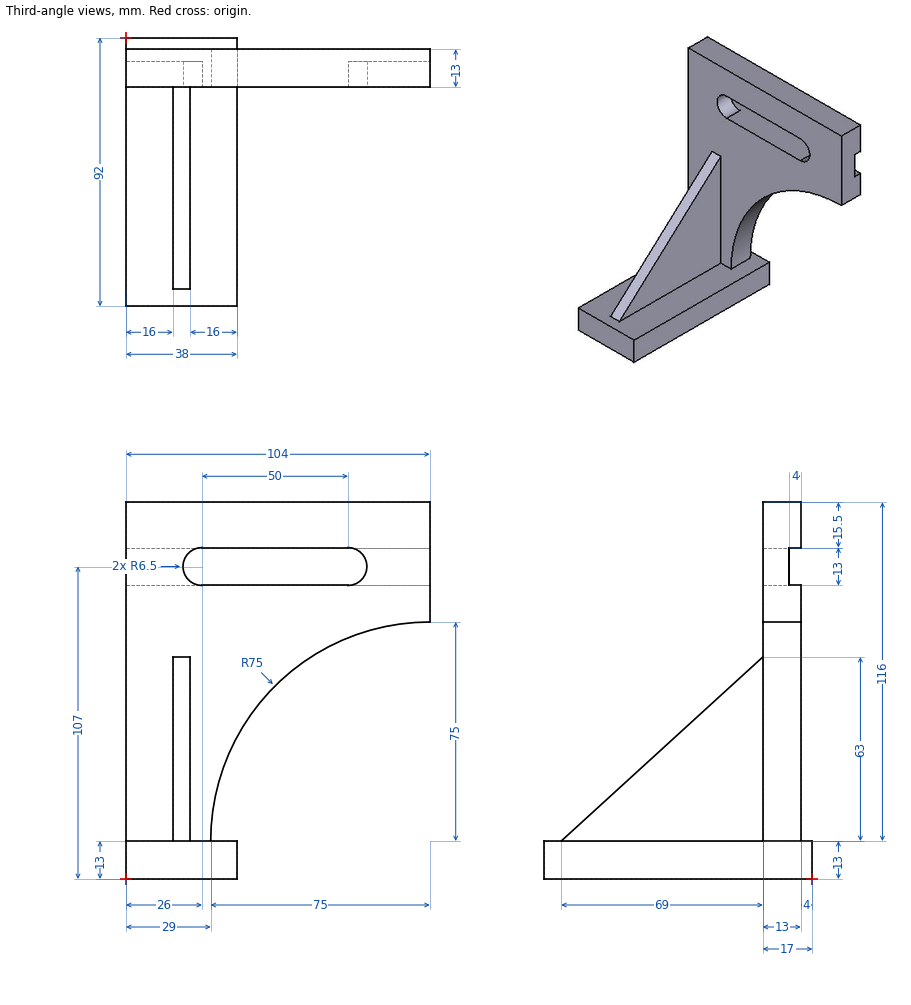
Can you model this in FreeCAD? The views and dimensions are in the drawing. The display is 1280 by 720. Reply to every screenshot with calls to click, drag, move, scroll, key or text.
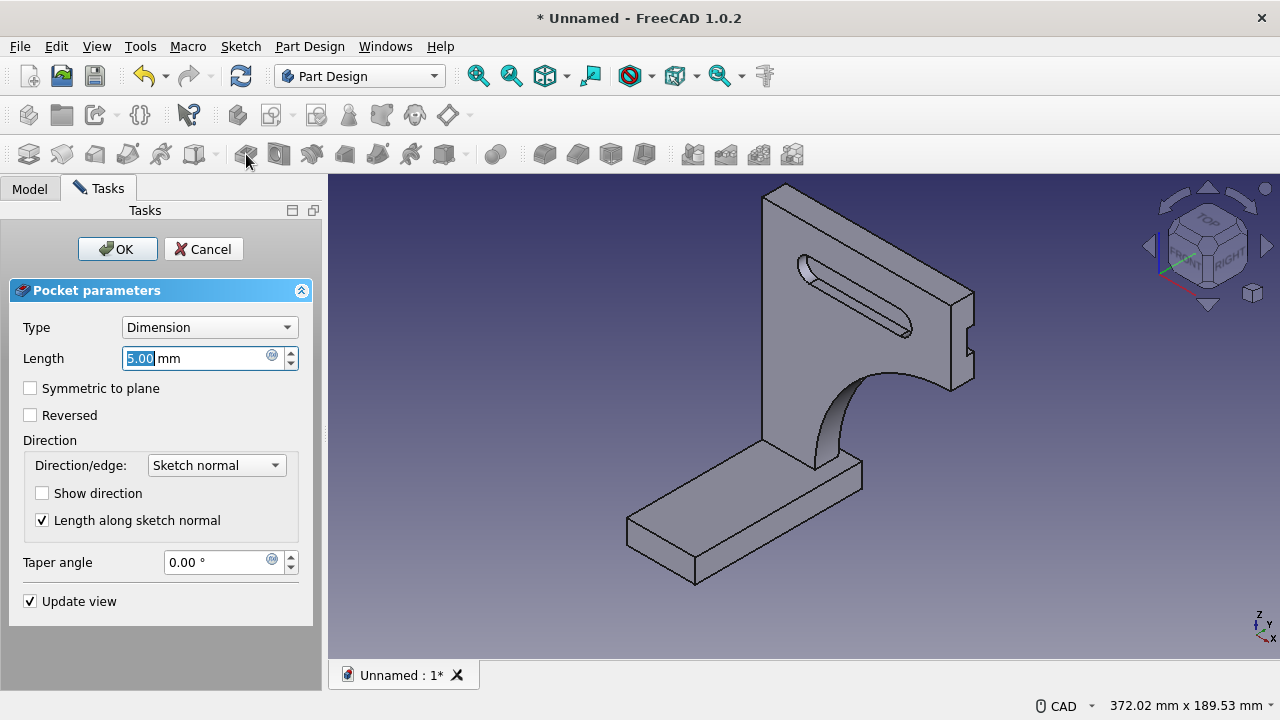
text(13)
key(Tab)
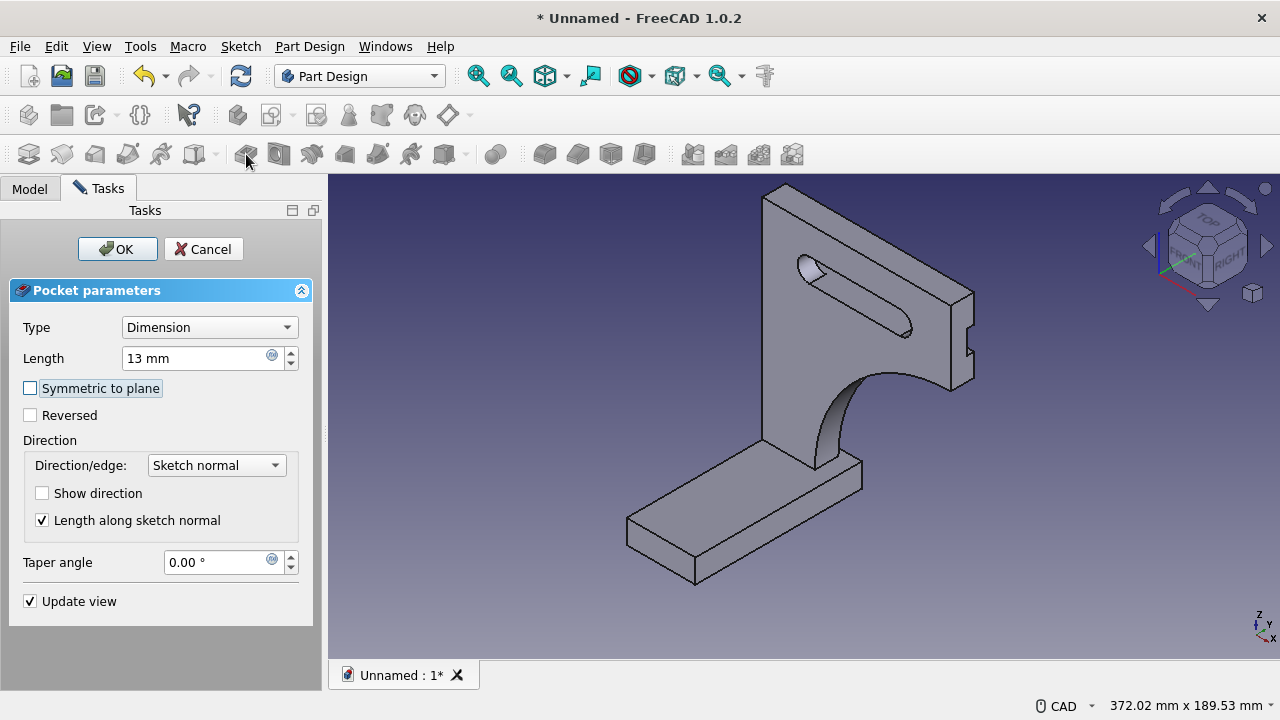
click(118, 249)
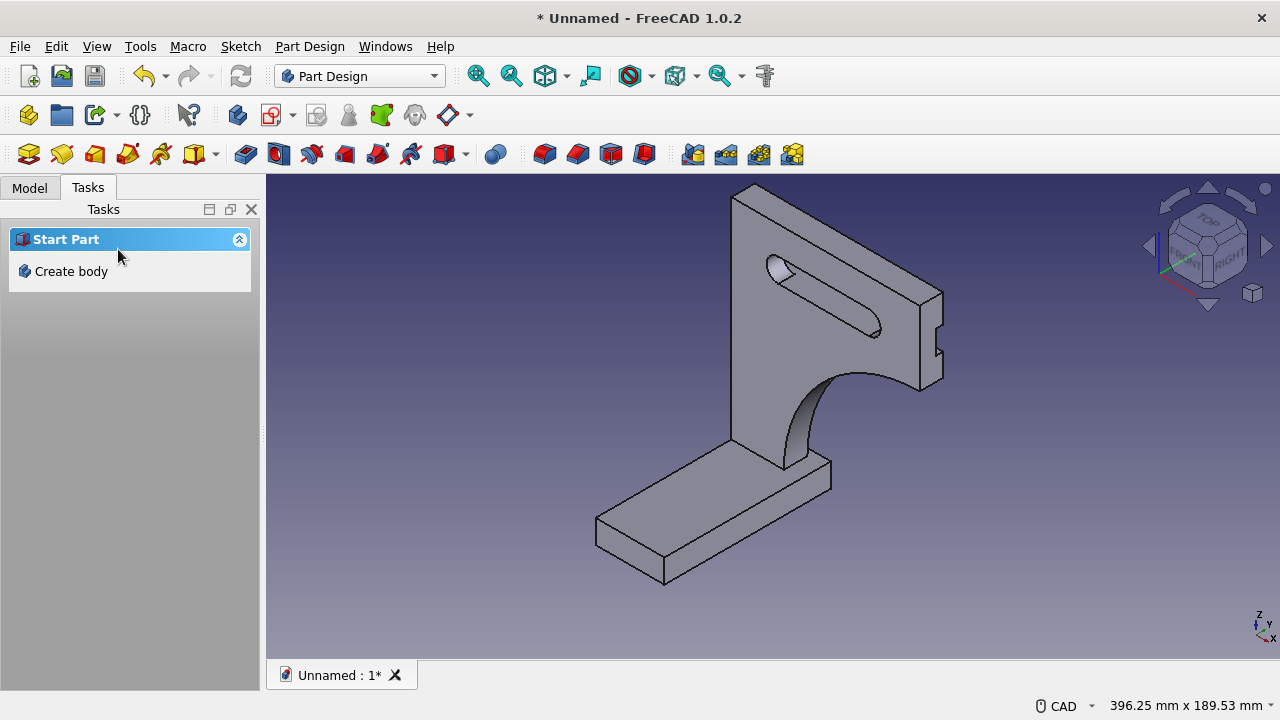
click(270, 116)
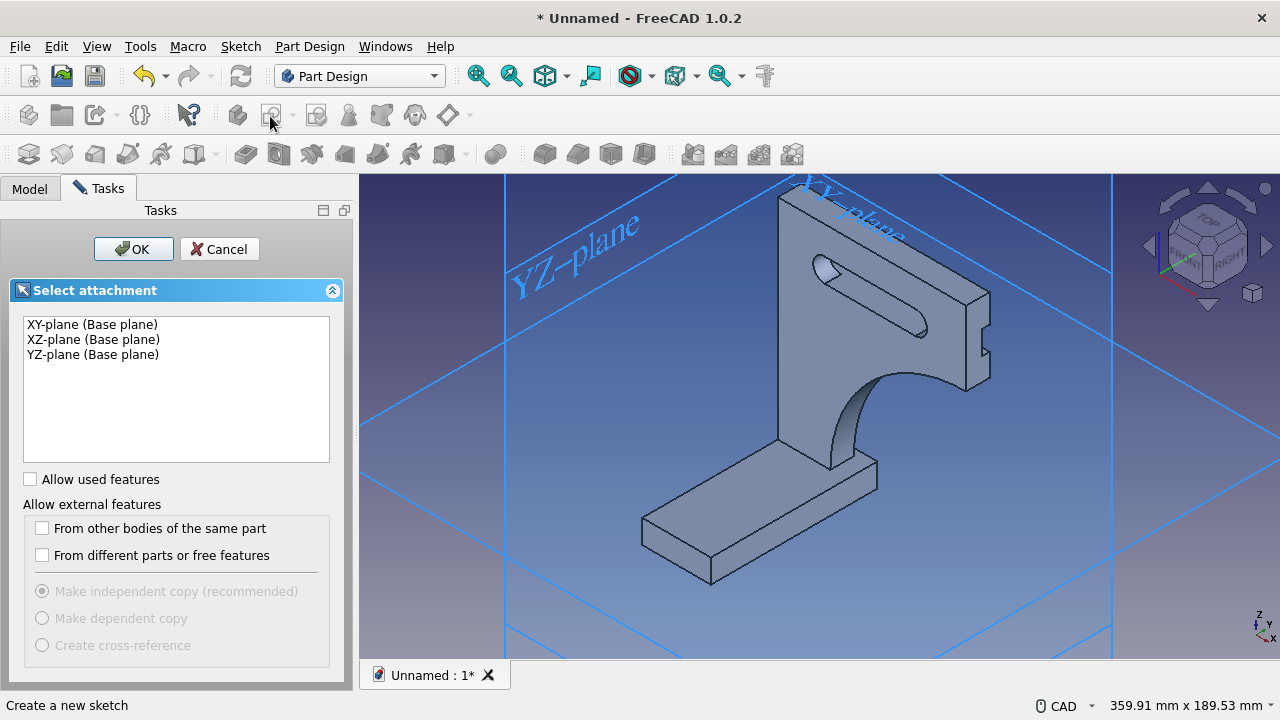
click(84, 354)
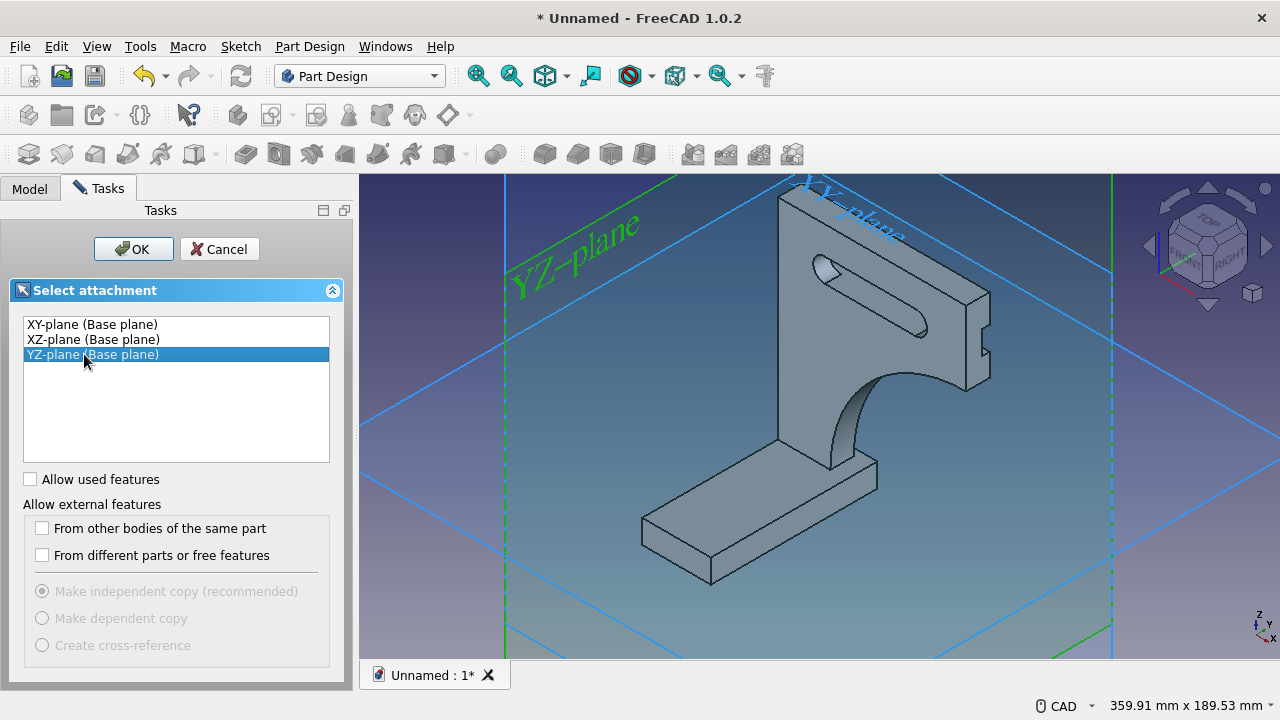
click(134, 249)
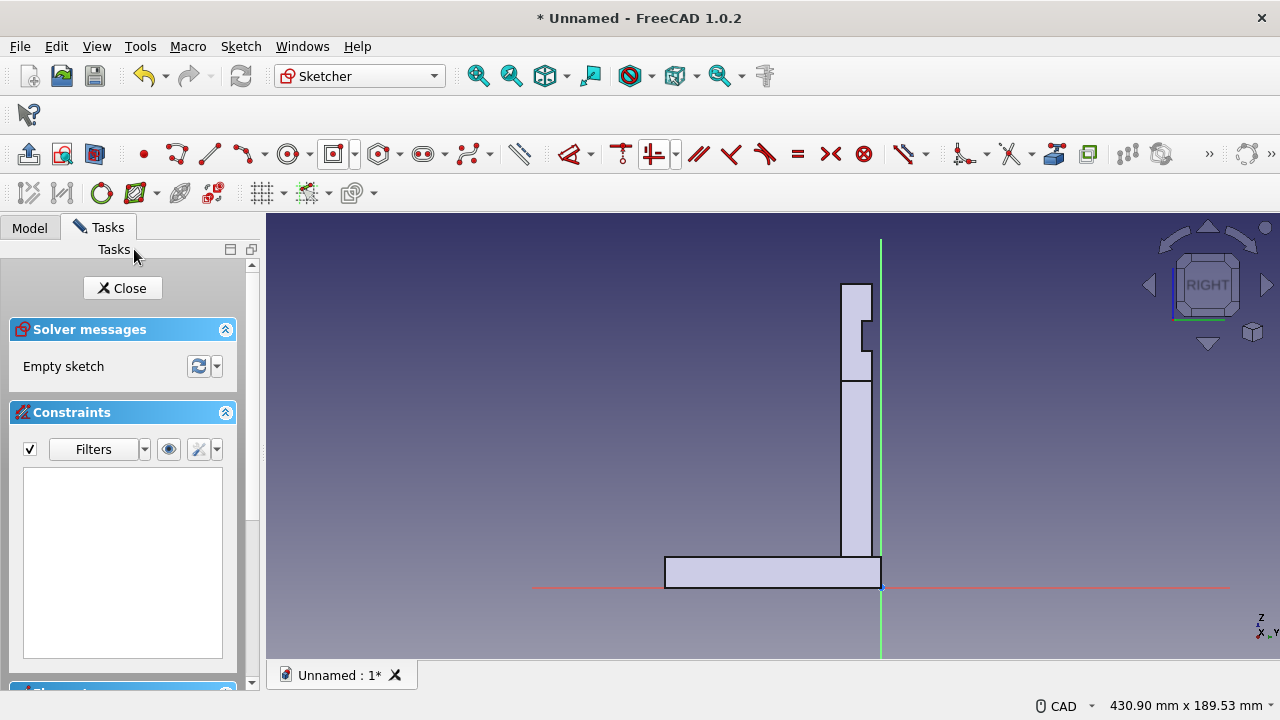
click(95, 154)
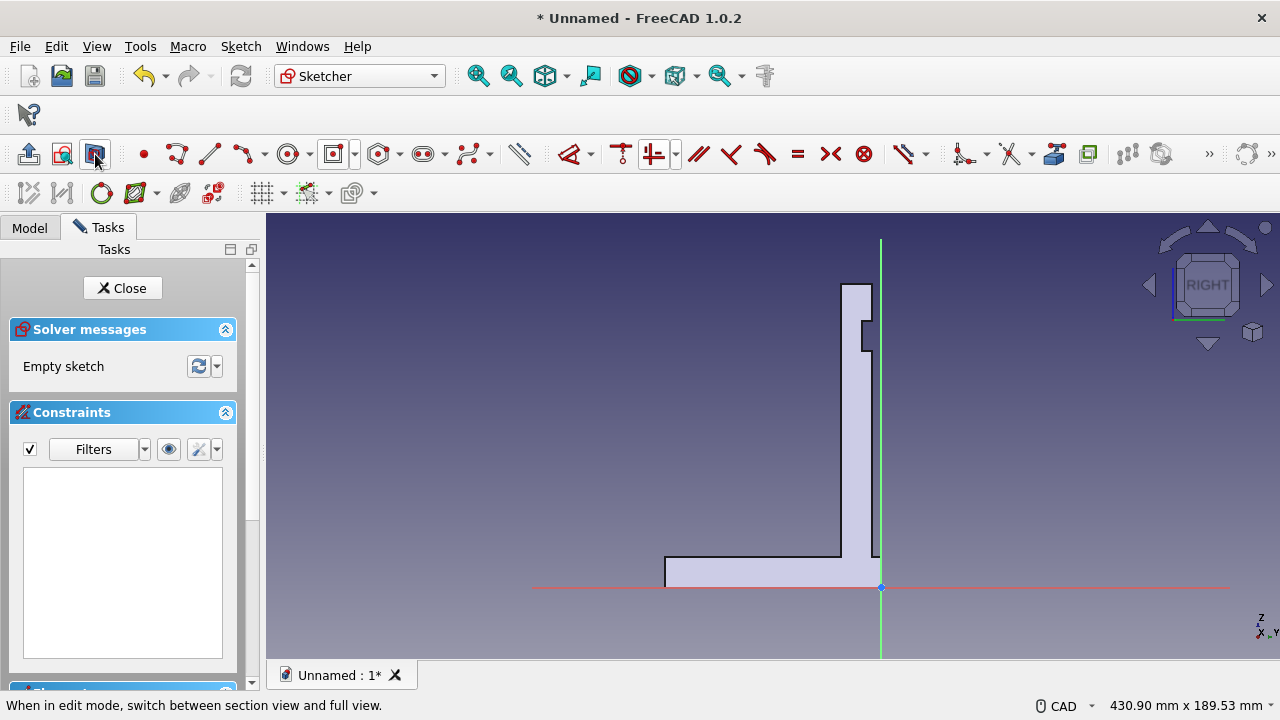
scroll(934, 625, up, 2)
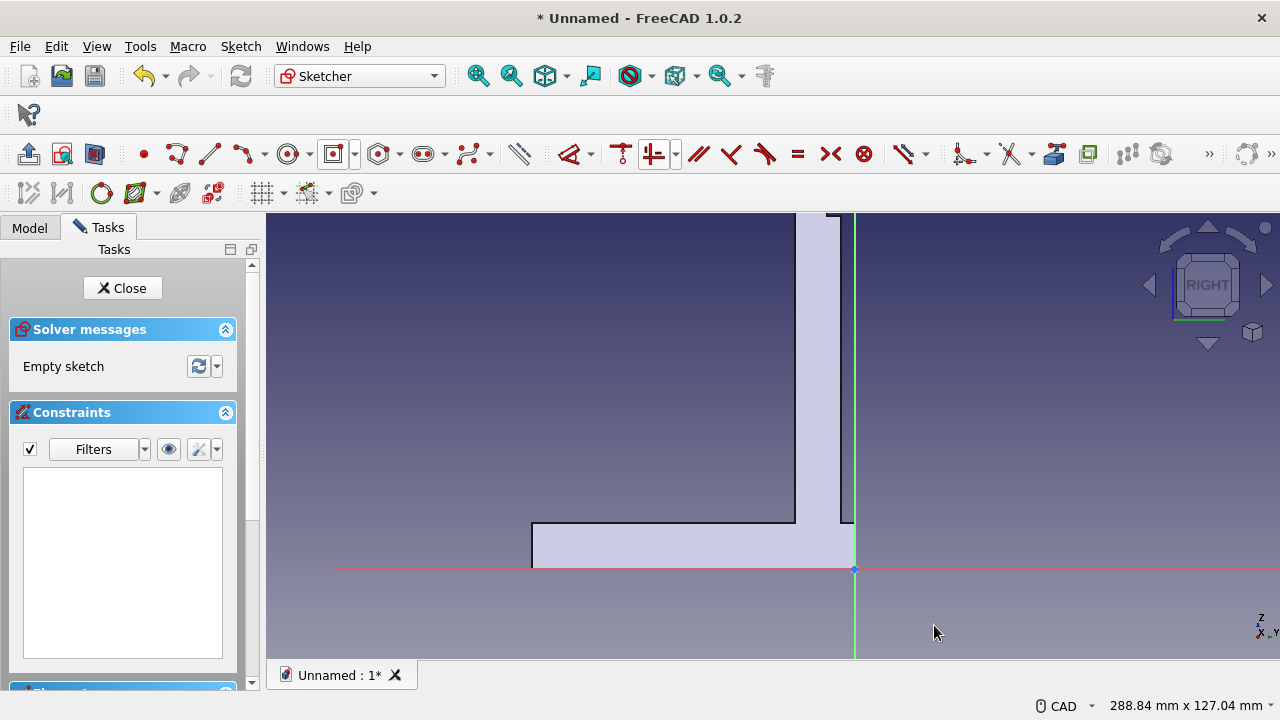
click(177, 154)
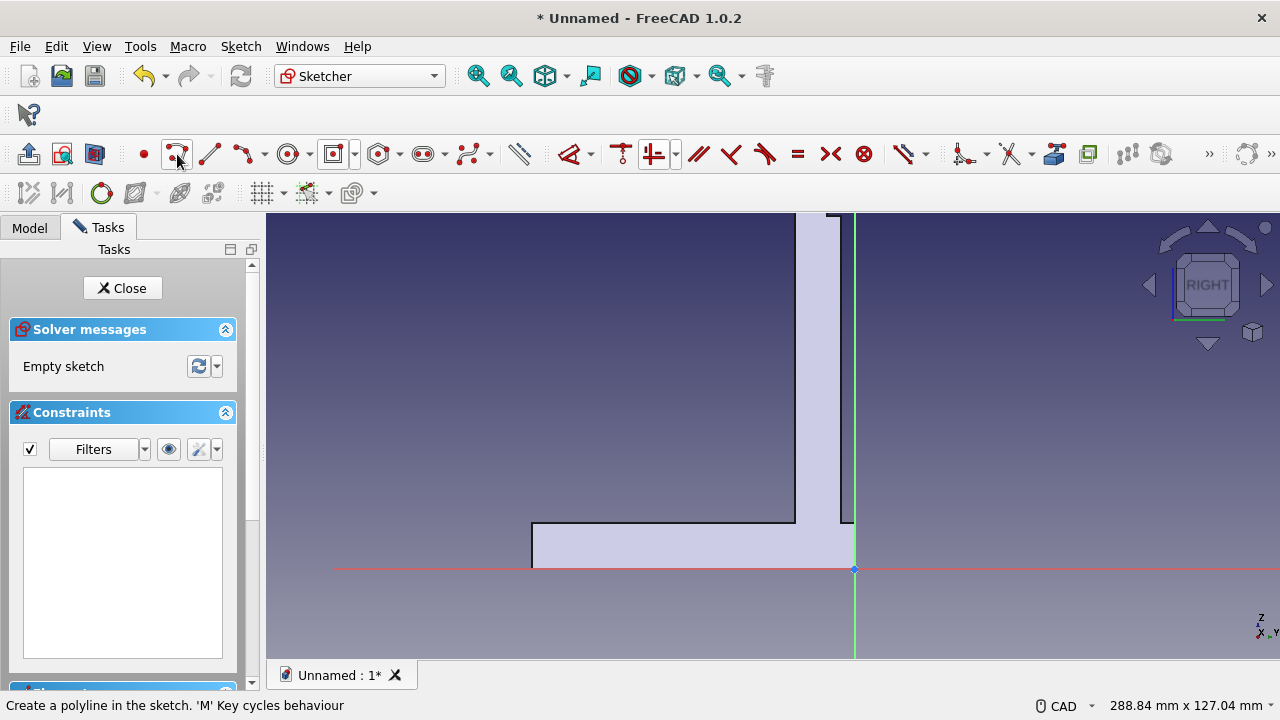
click(795, 523)
click(553, 523)
click(795, 302)
click(795, 524)
key(Escape)
key(Escape)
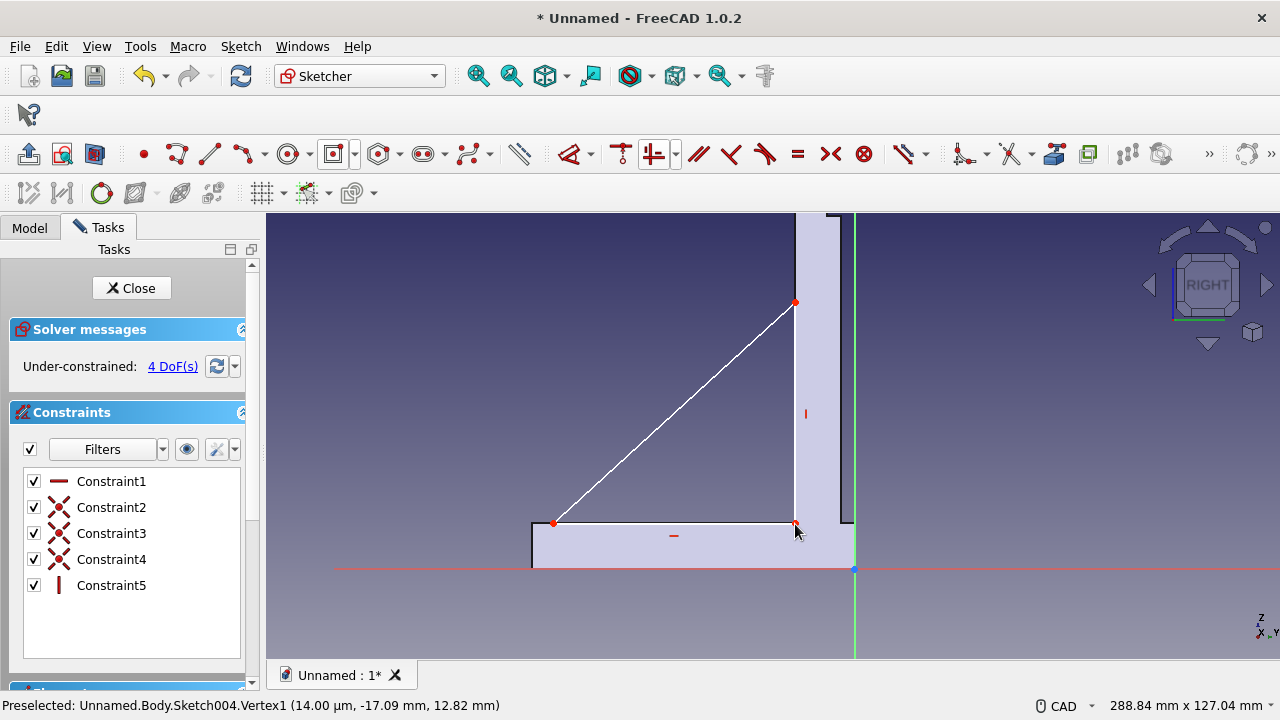
click(568, 154)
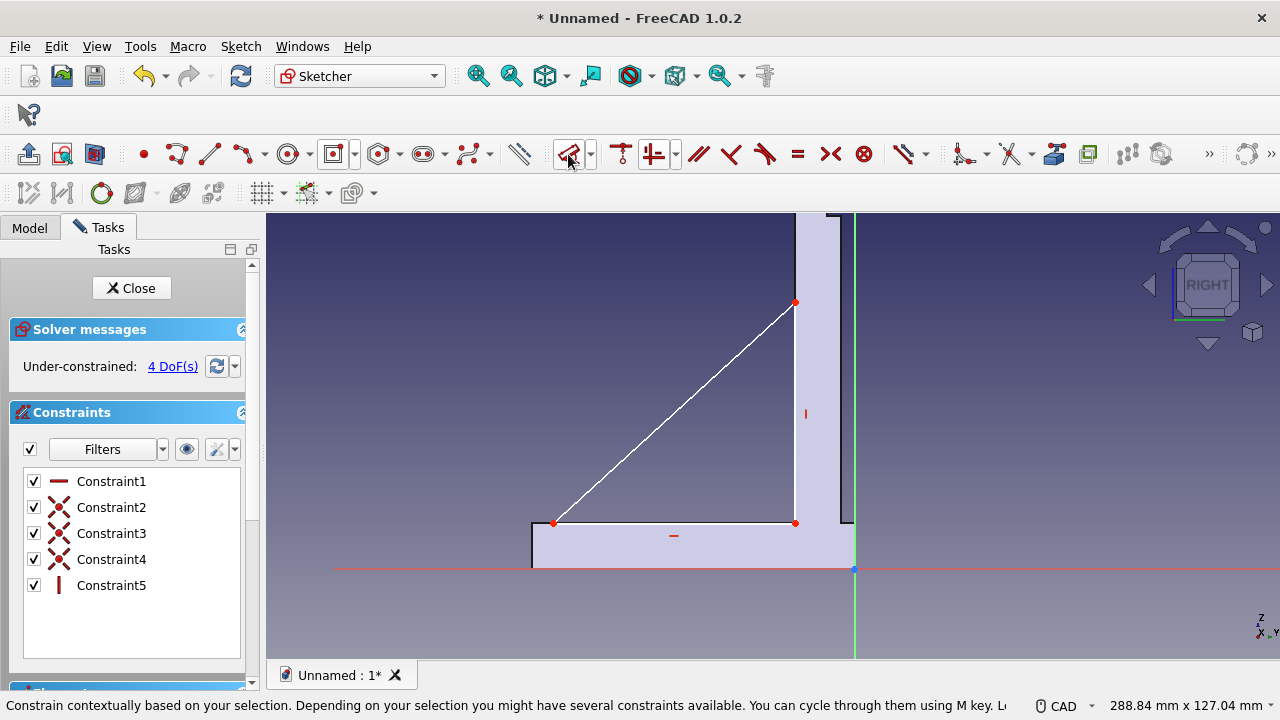
click(722, 524)
click(674, 490)